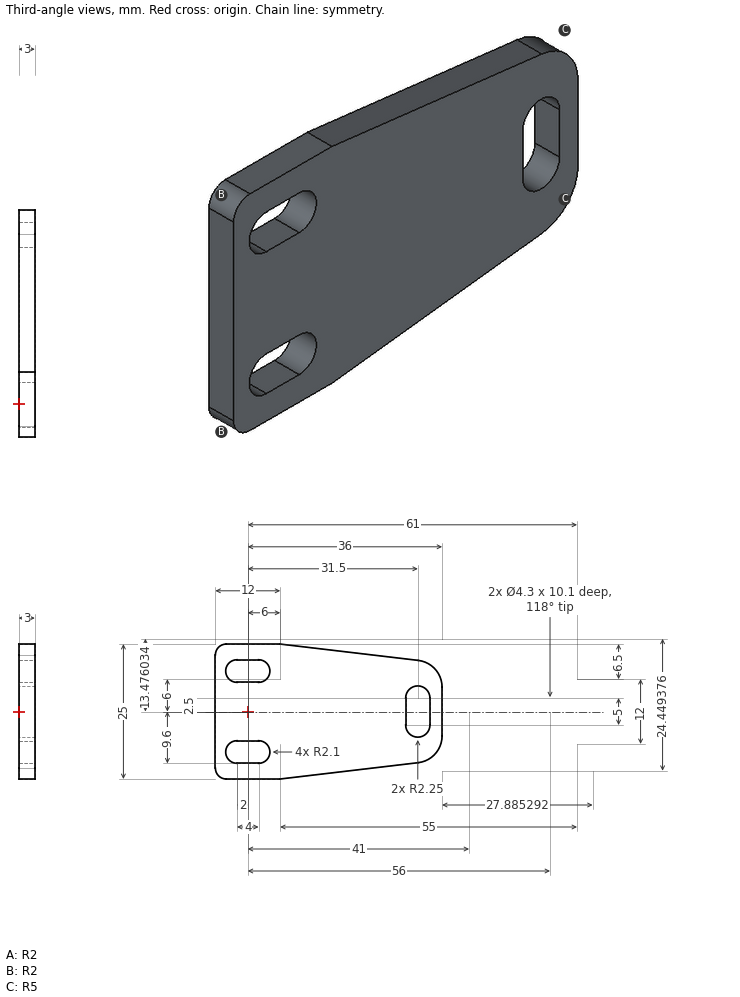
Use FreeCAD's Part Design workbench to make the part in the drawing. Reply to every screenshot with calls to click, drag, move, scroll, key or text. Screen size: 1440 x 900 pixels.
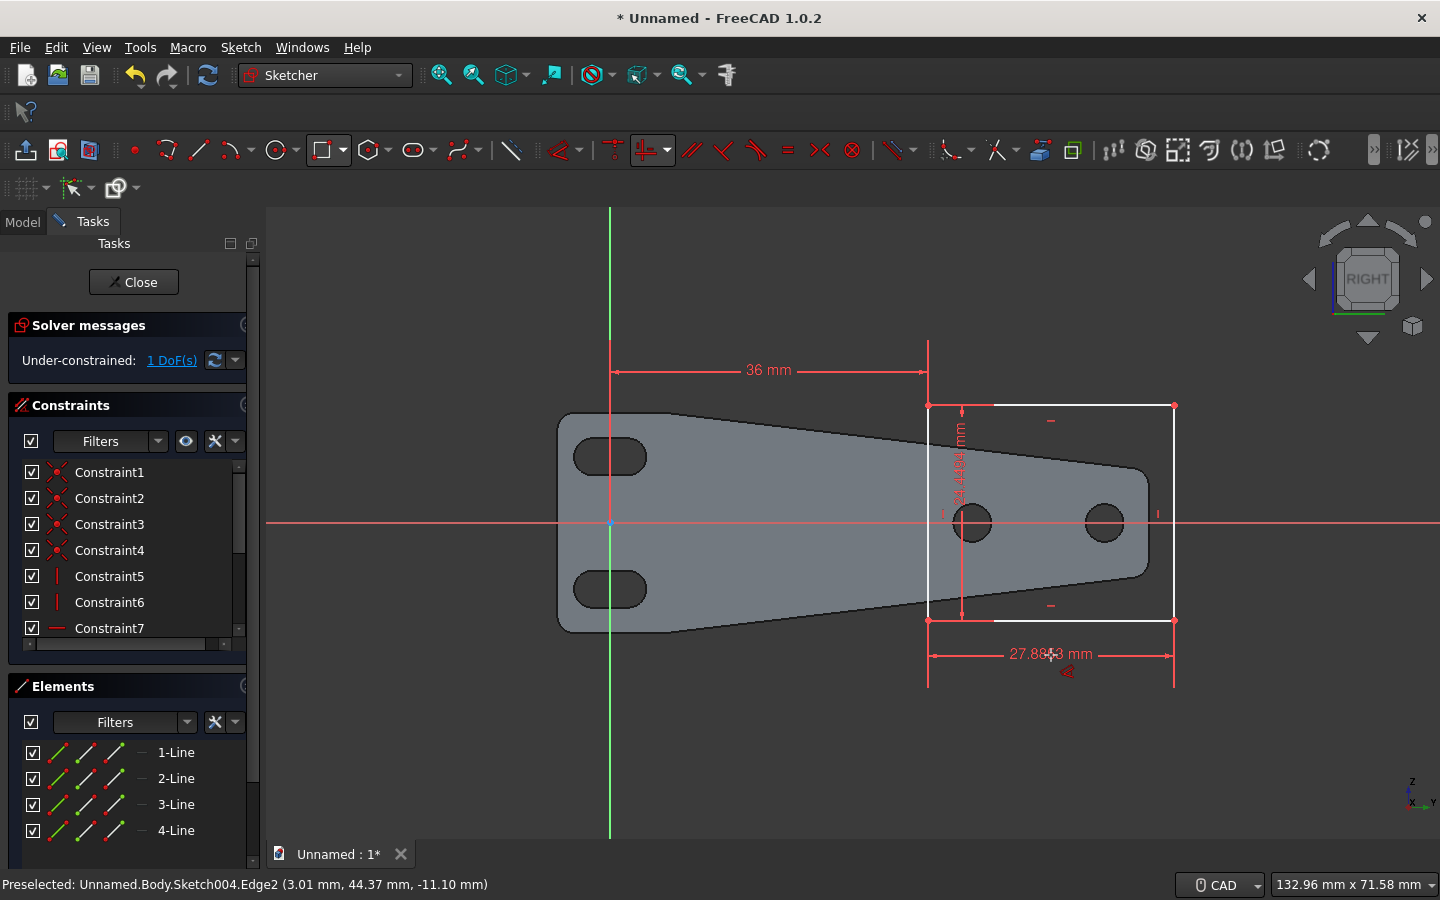
click(928, 405)
click(576, 464)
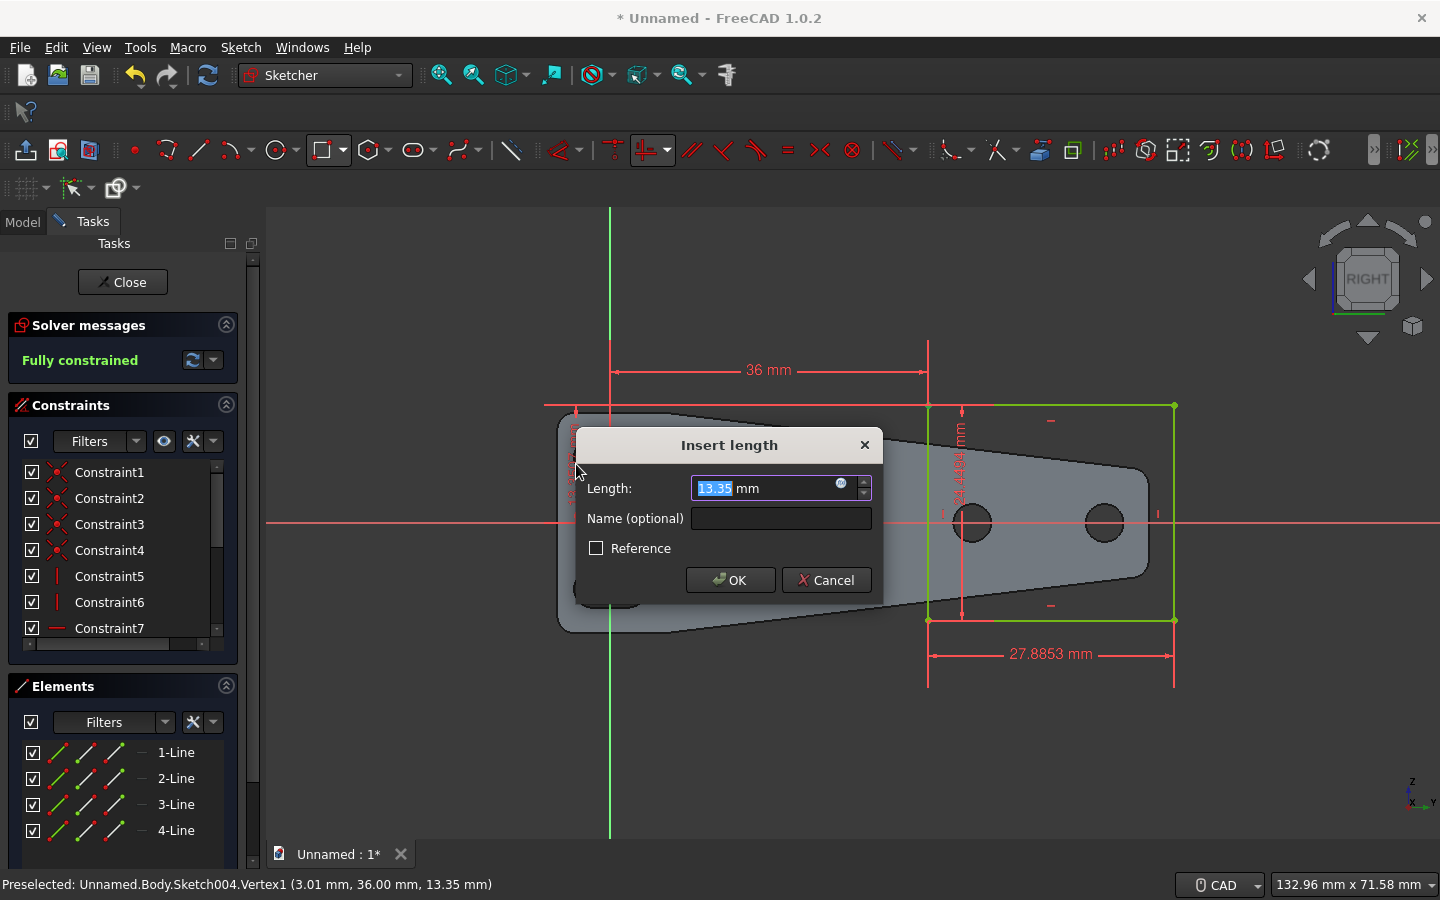
text(13.476034)
key(Return)
key(Escape)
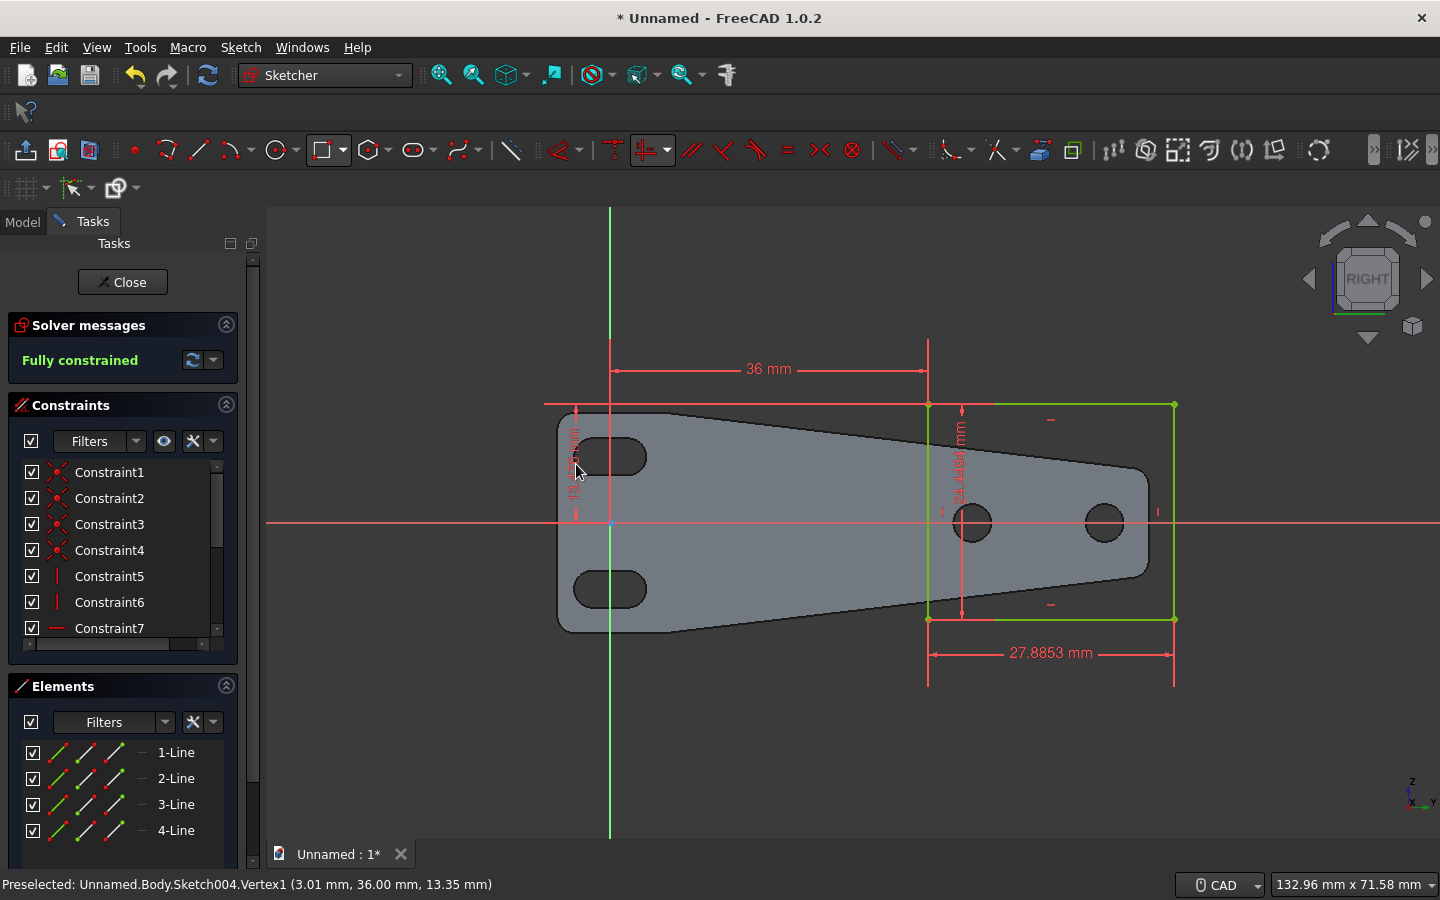
click(123, 282)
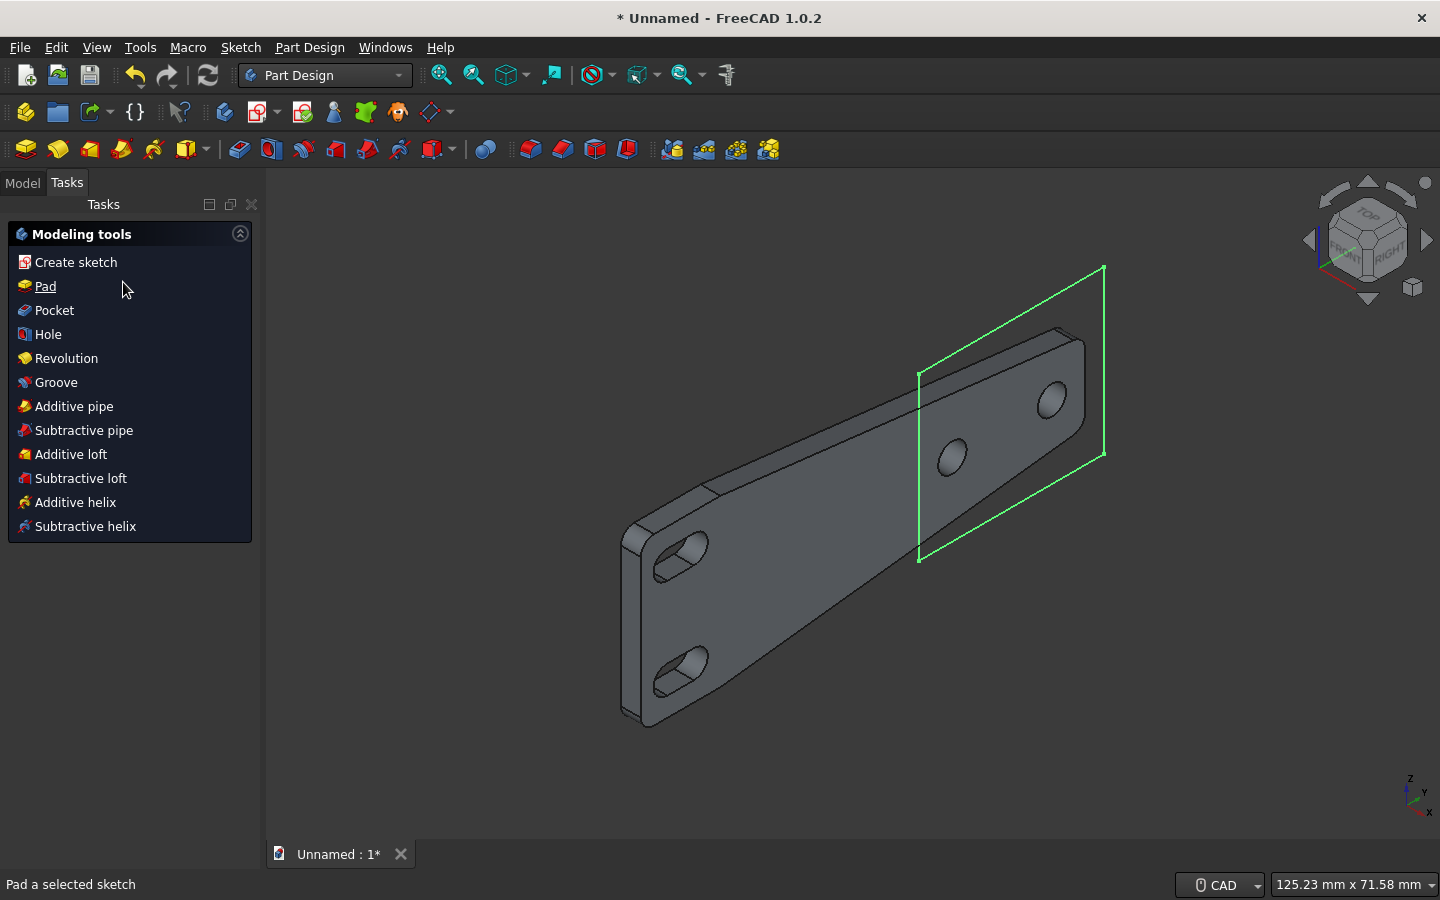
click(240, 150)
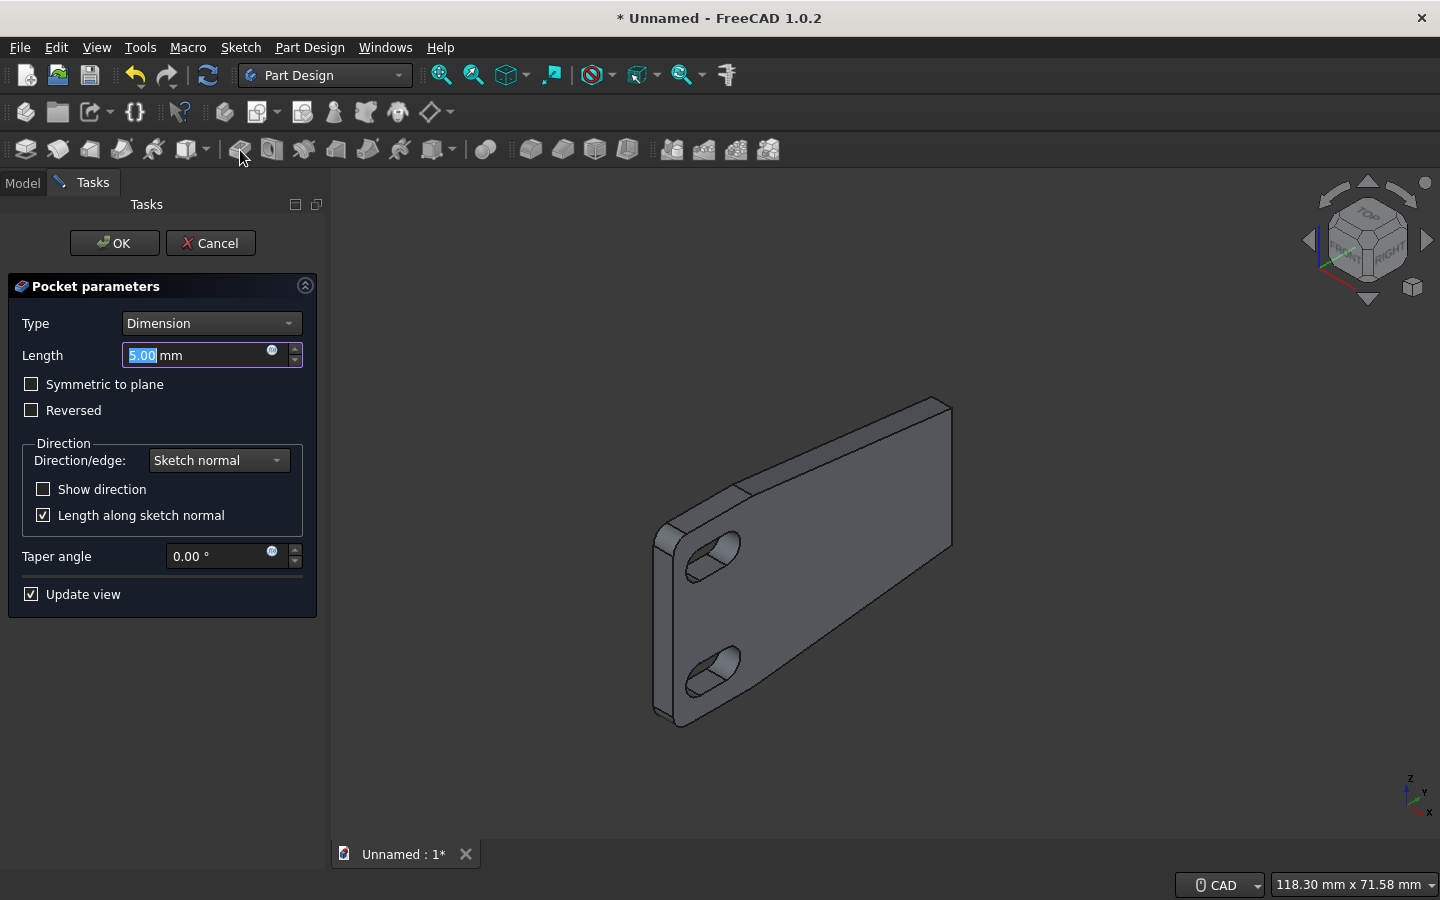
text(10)
key(Tab)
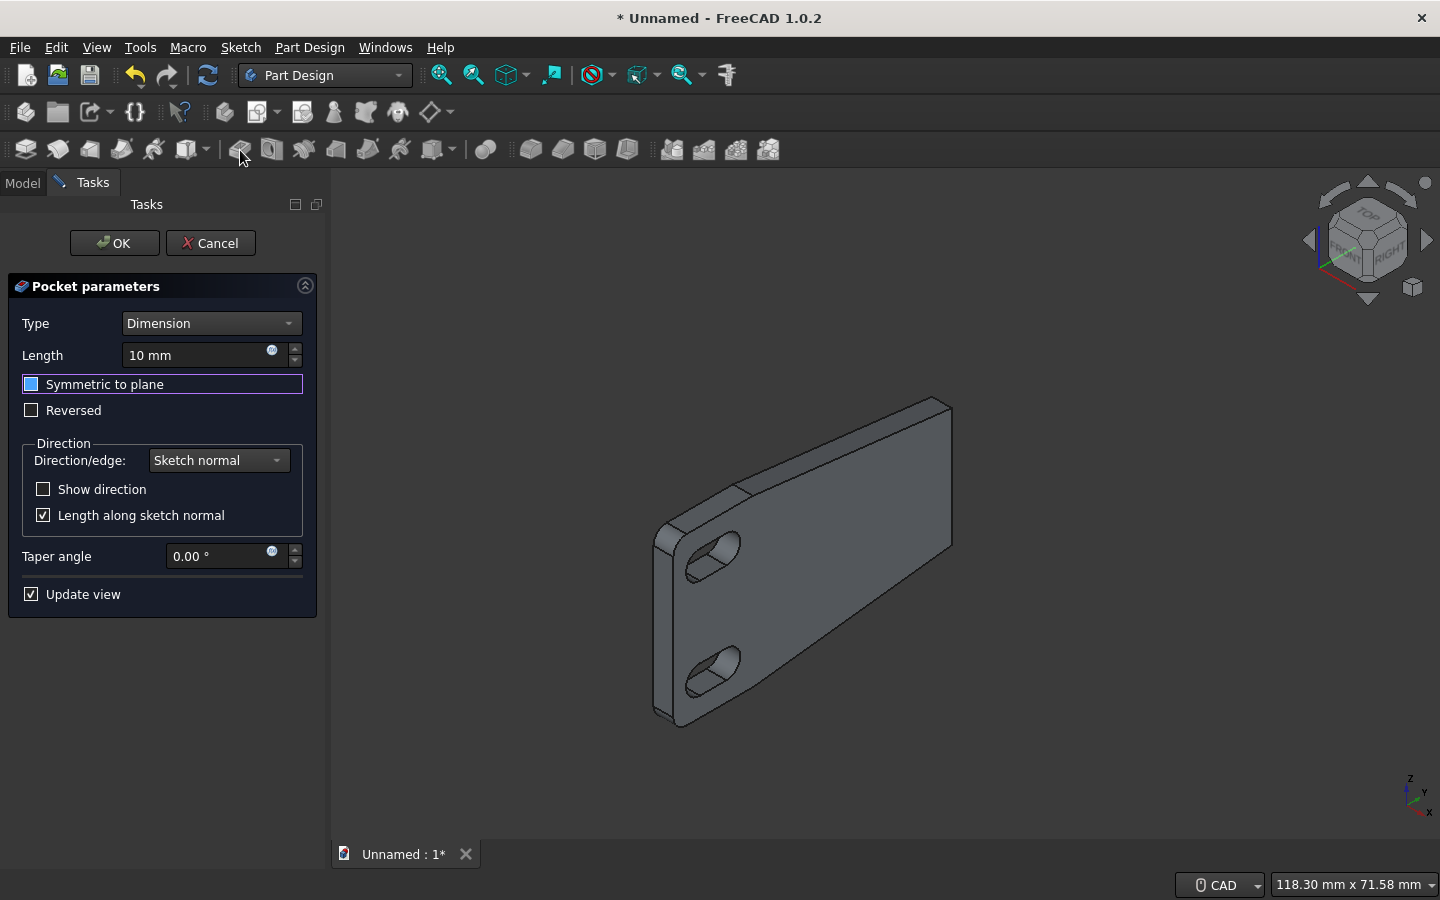
click(115, 243)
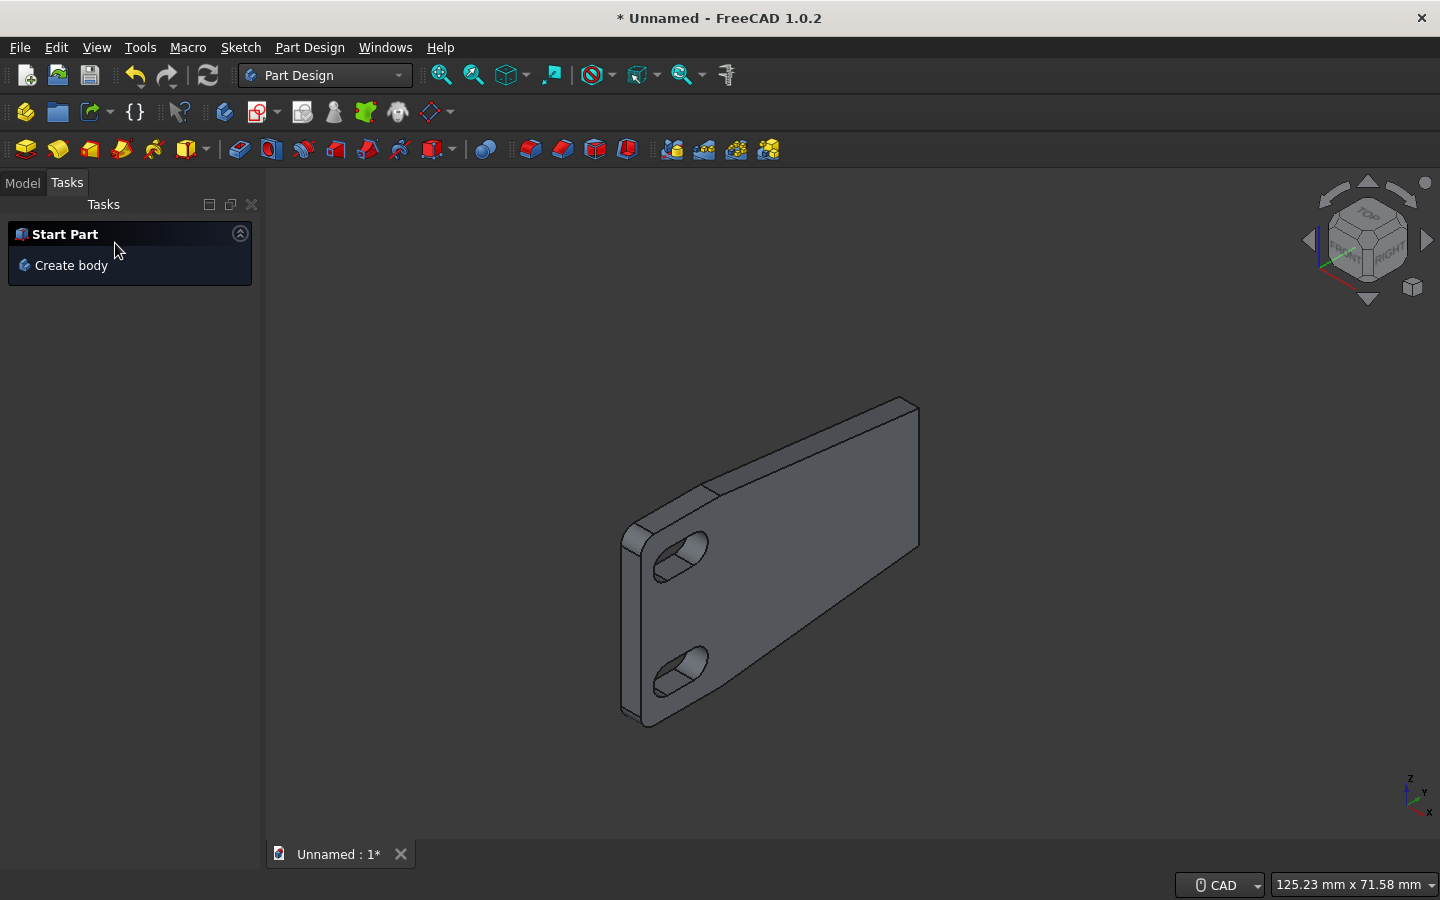
key(6)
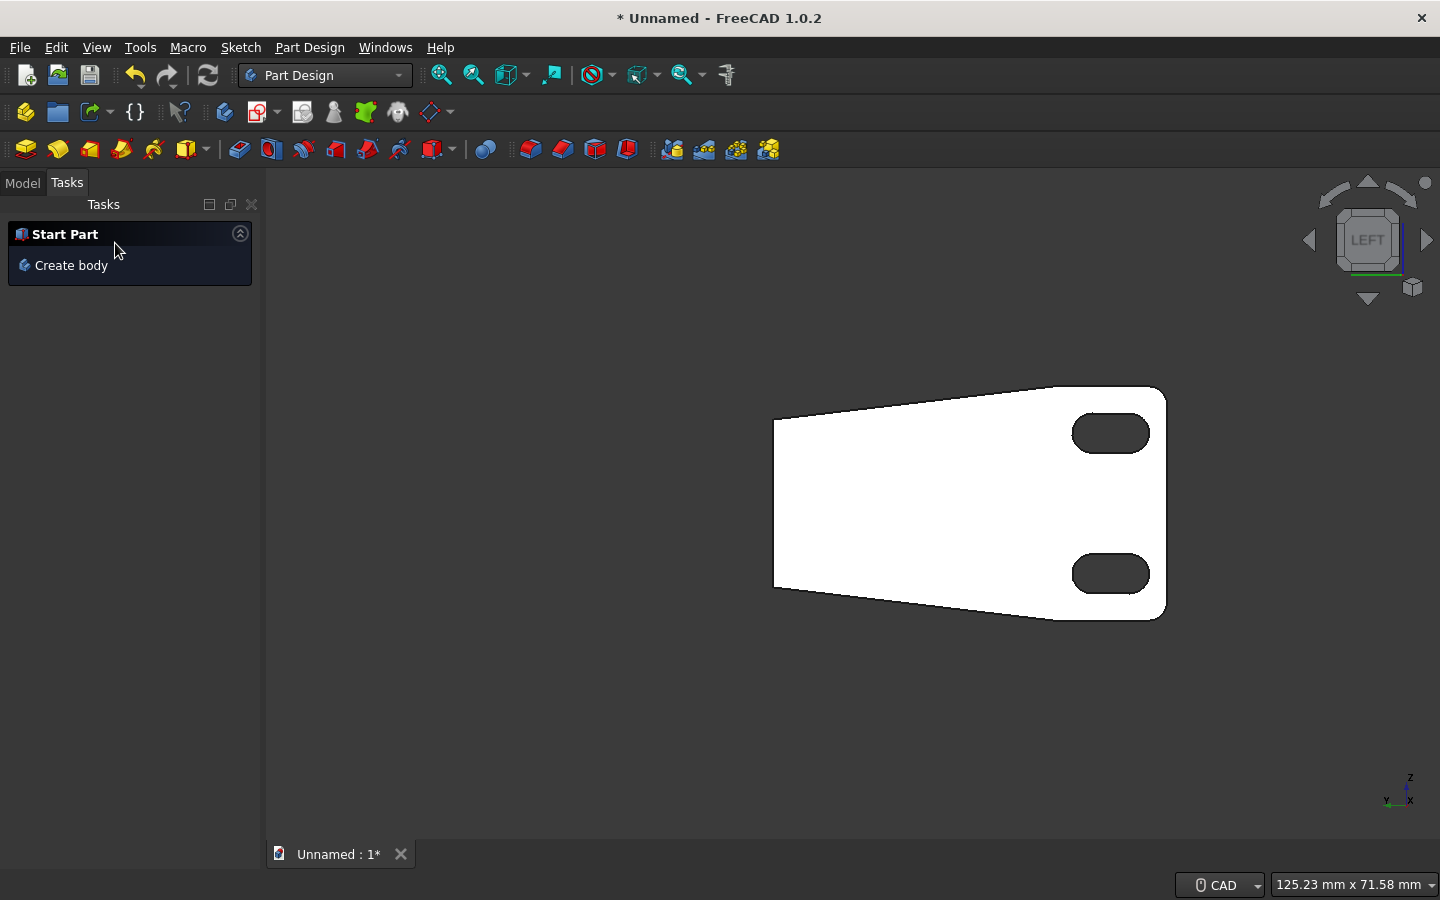
key(v)
key(f)